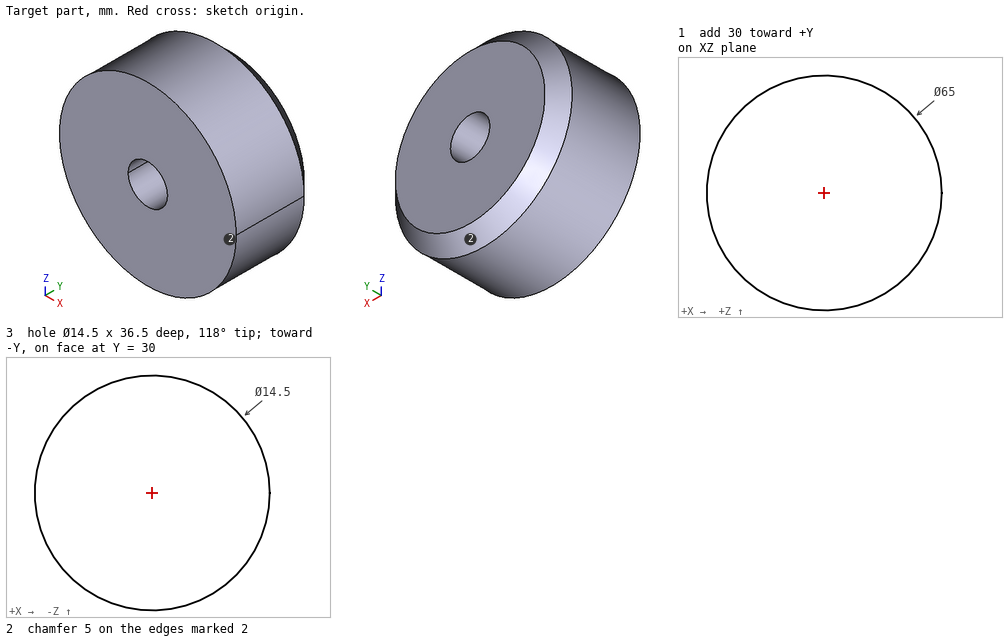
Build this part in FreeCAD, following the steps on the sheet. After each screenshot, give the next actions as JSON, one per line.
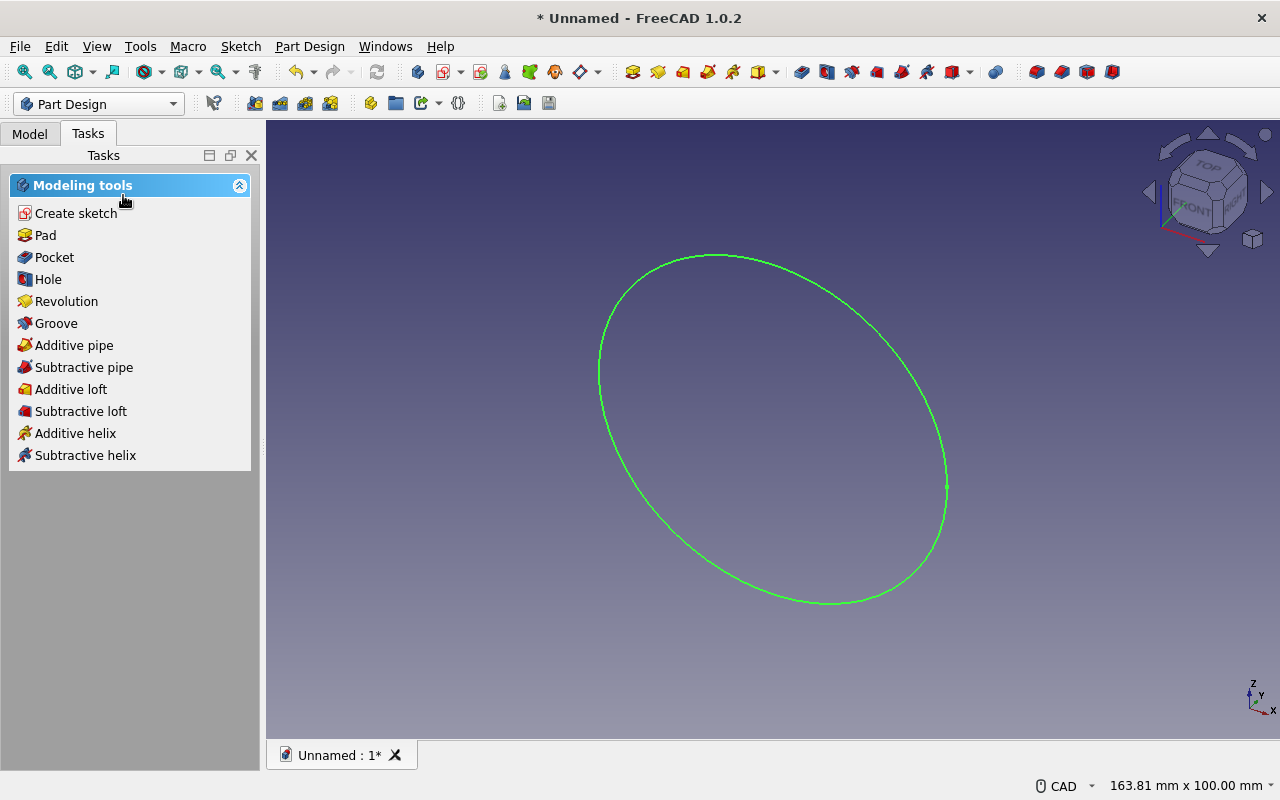
{"action": "left_click", "coordinate": [633, 72]}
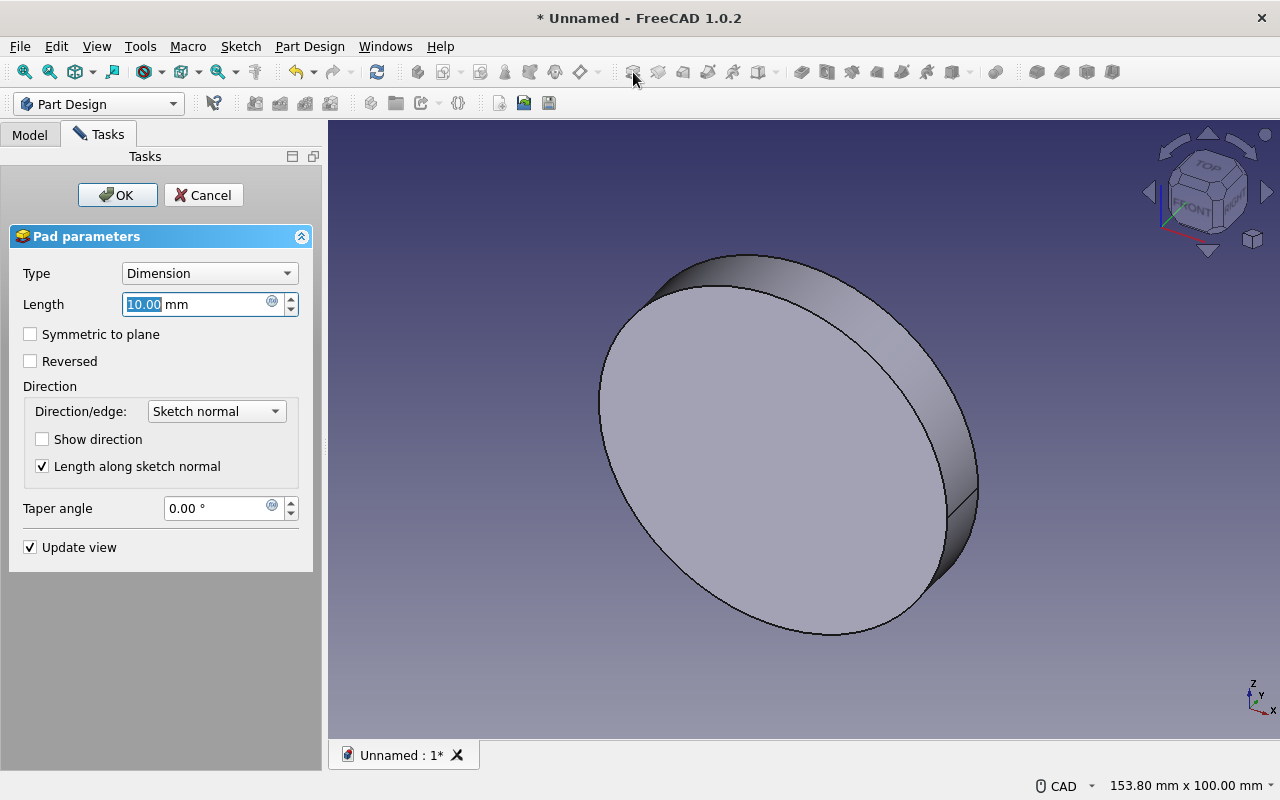
{"action": "type", "text": "30"}
{"action": "key", "text": "Tab"}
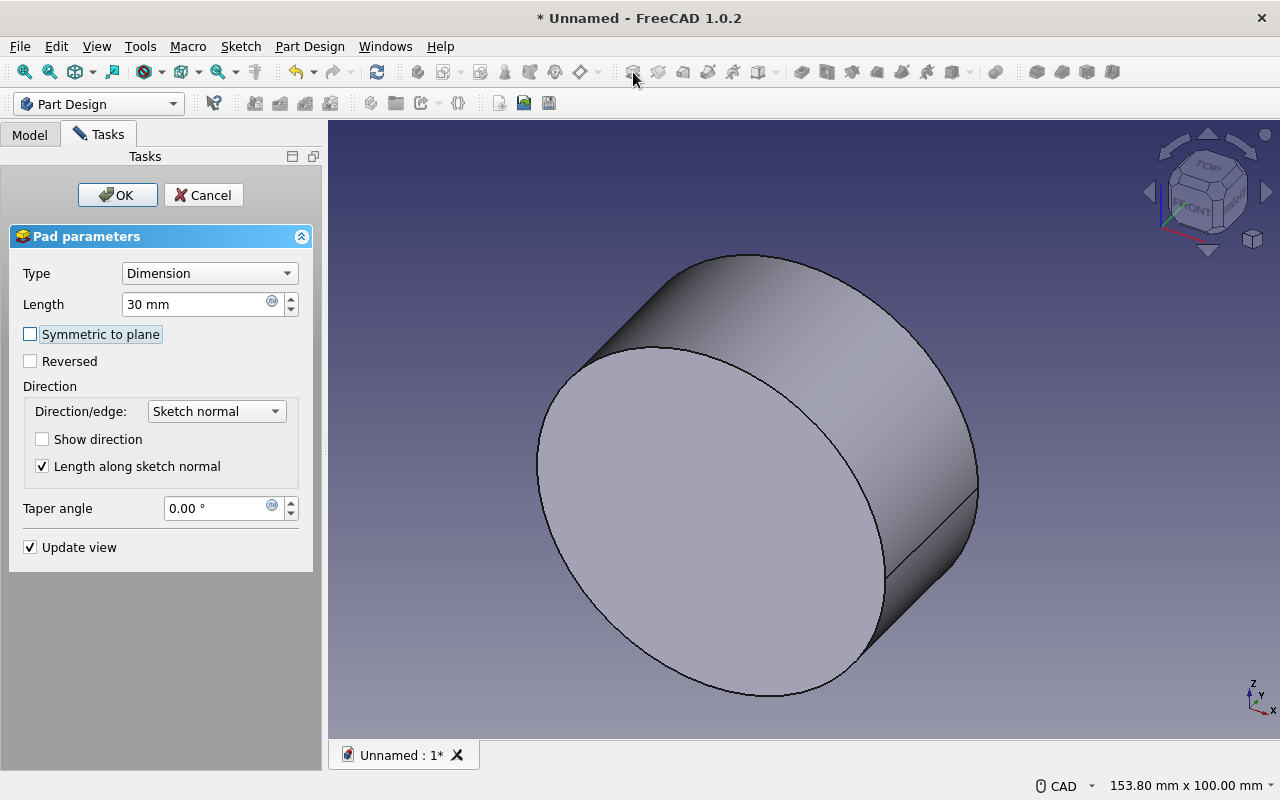
{"action": "left_click", "coordinate": [31, 361]}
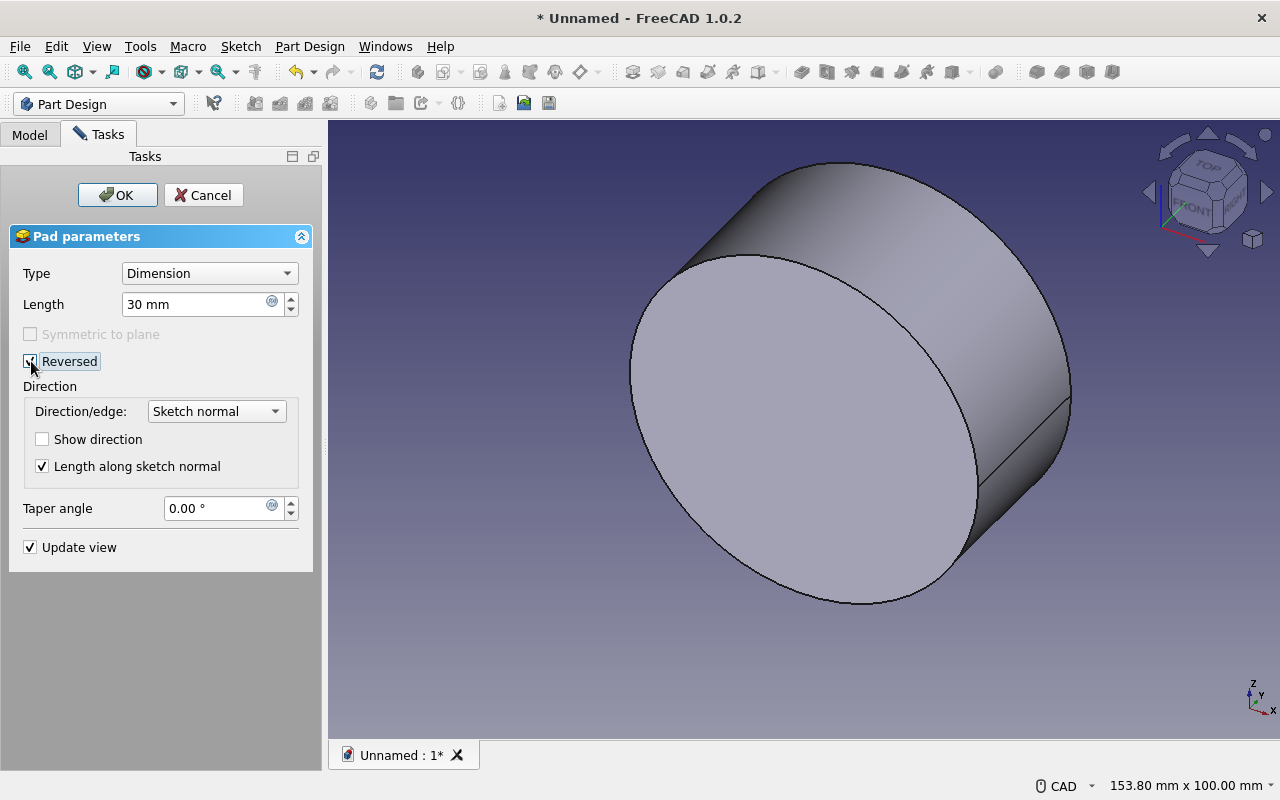
{"action": "left_click", "coordinate": [118, 195]}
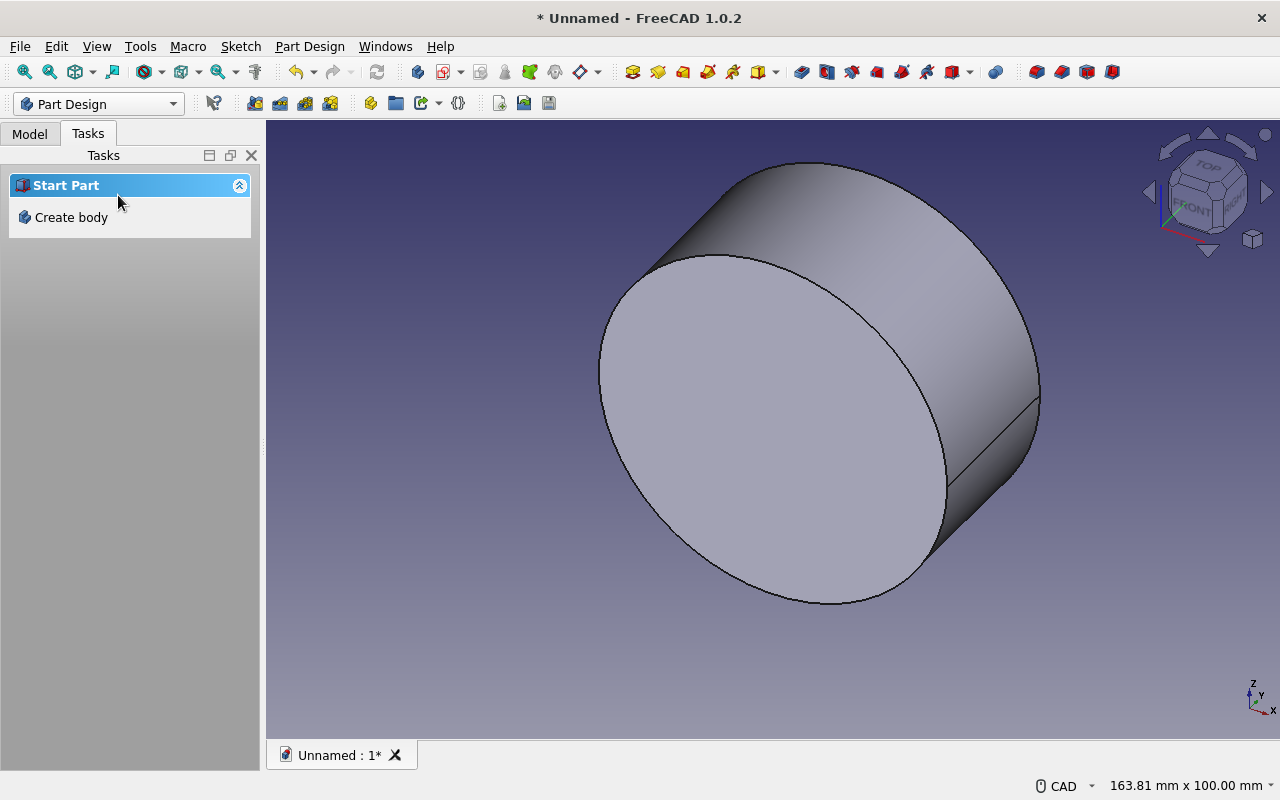
{"action": "left_click", "coordinate": [25, 72]}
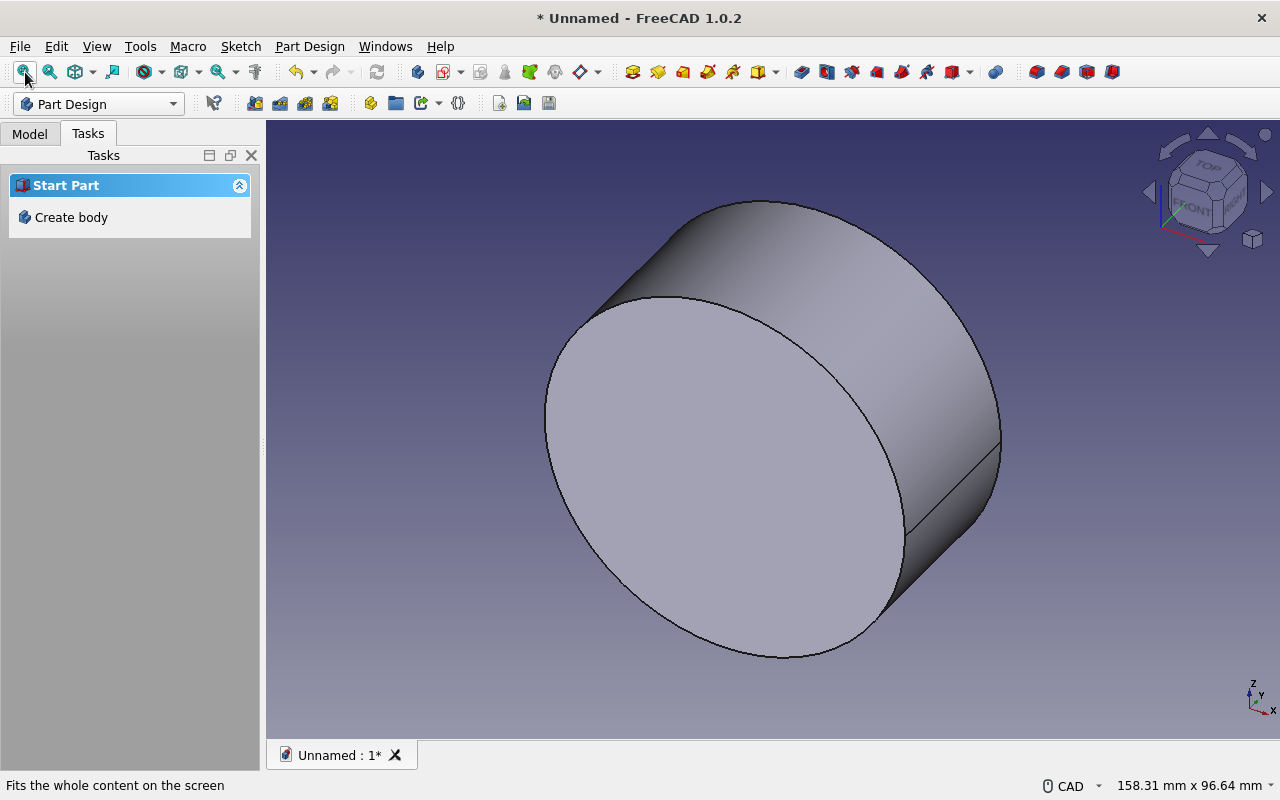
{"action": "key", "text": "0"}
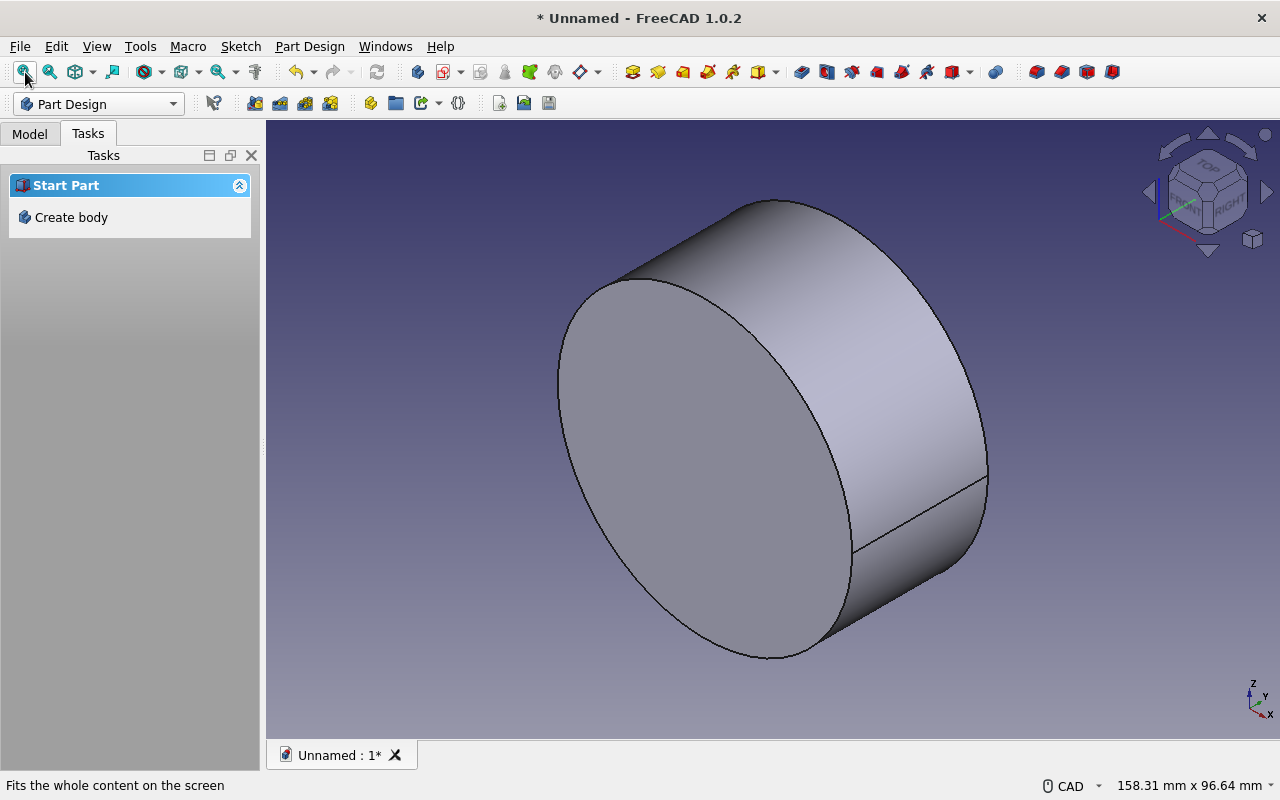
{"action": "key", "text": "2"}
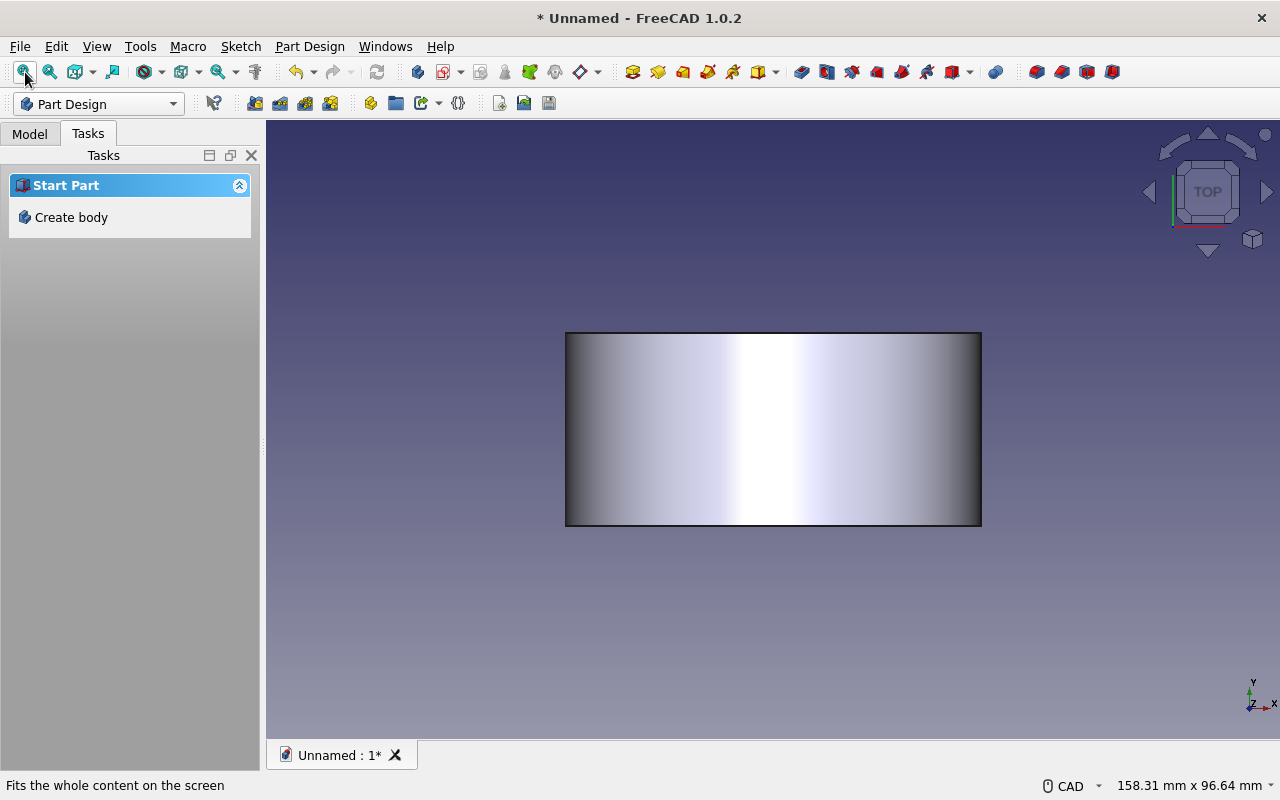
{"action": "left_click", "coordinate": [25, 72]}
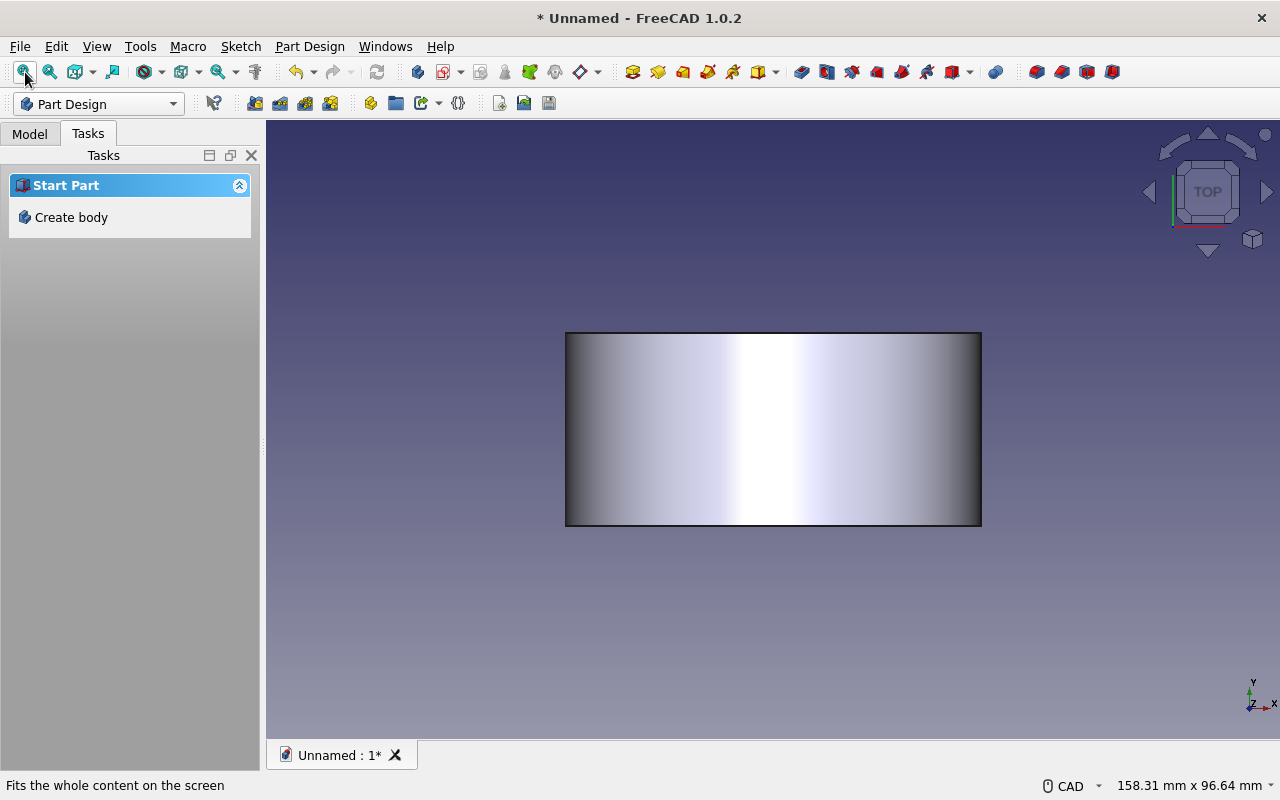
{"action": "left_click", "coordinate": [604, 332]}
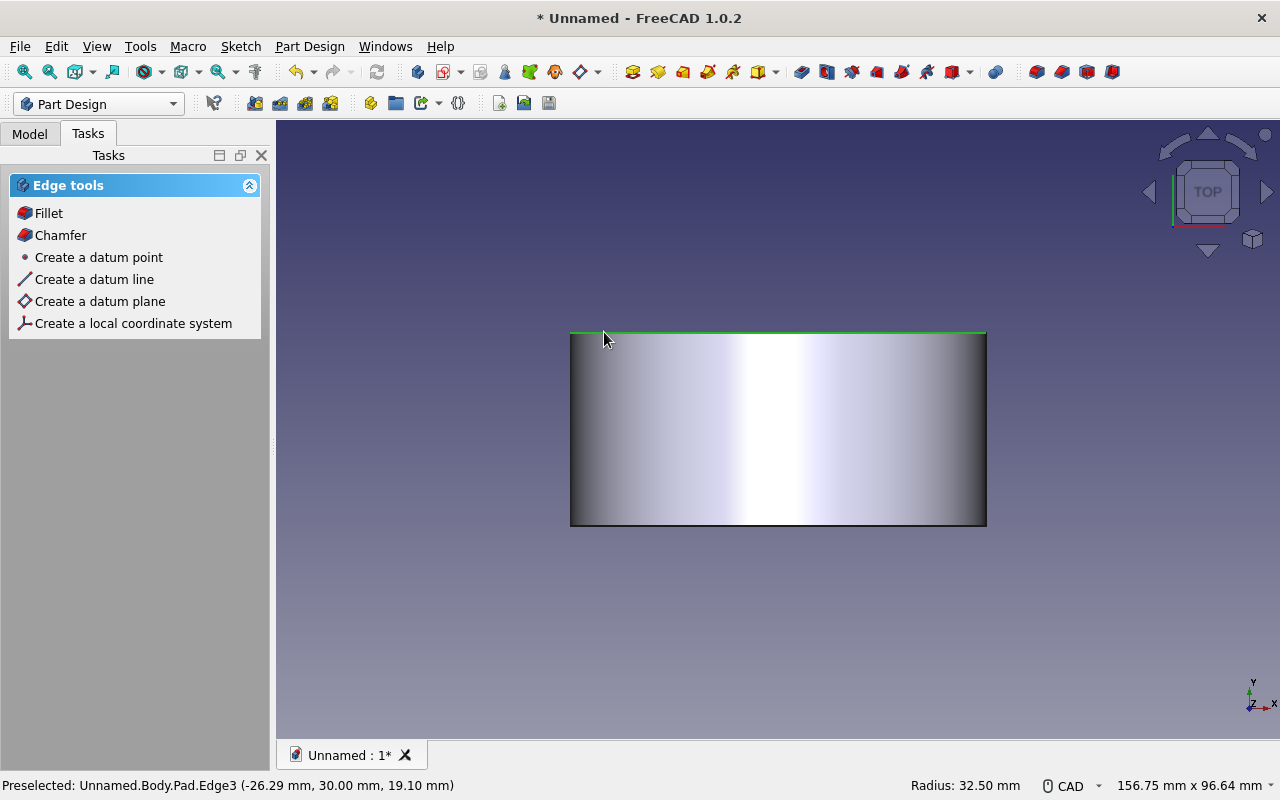
{"action": "left_click", "coordinate": [1062, 72]}